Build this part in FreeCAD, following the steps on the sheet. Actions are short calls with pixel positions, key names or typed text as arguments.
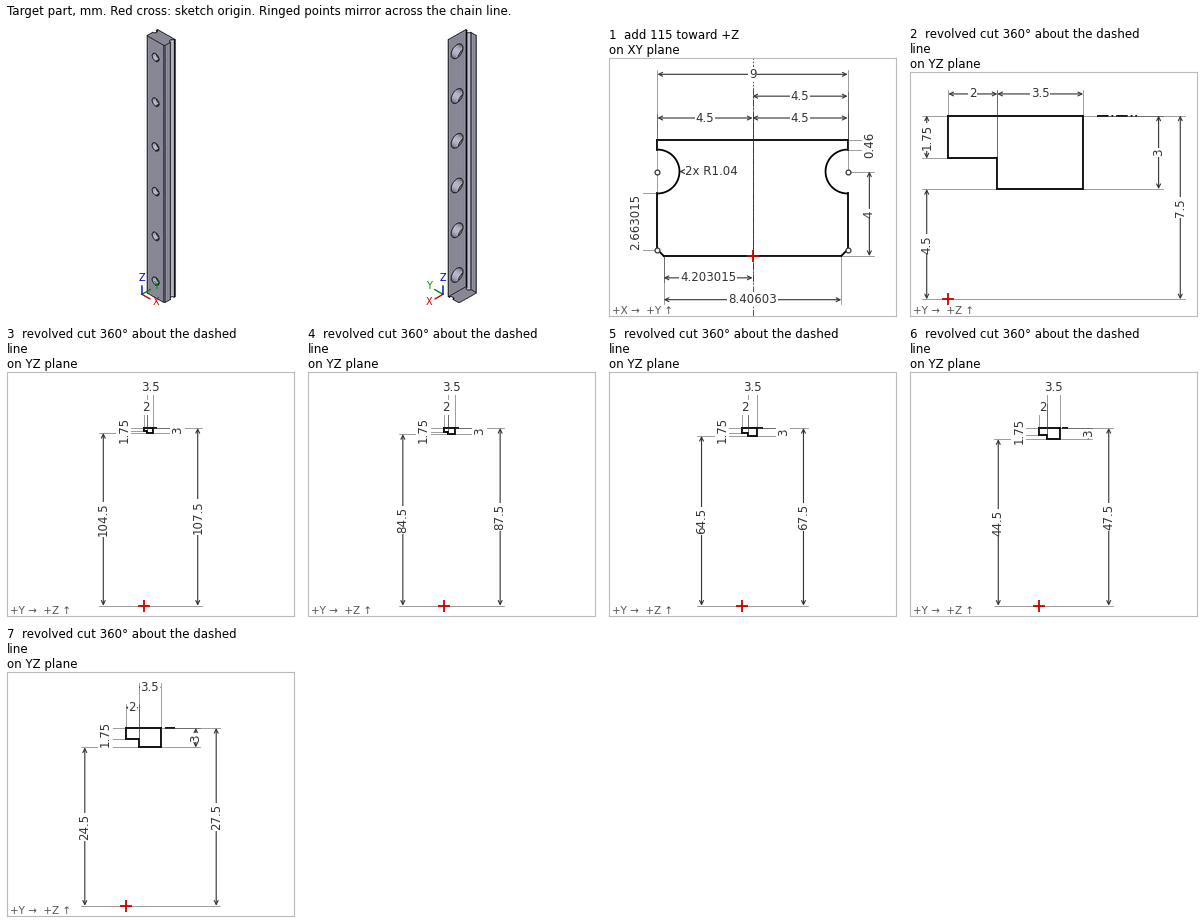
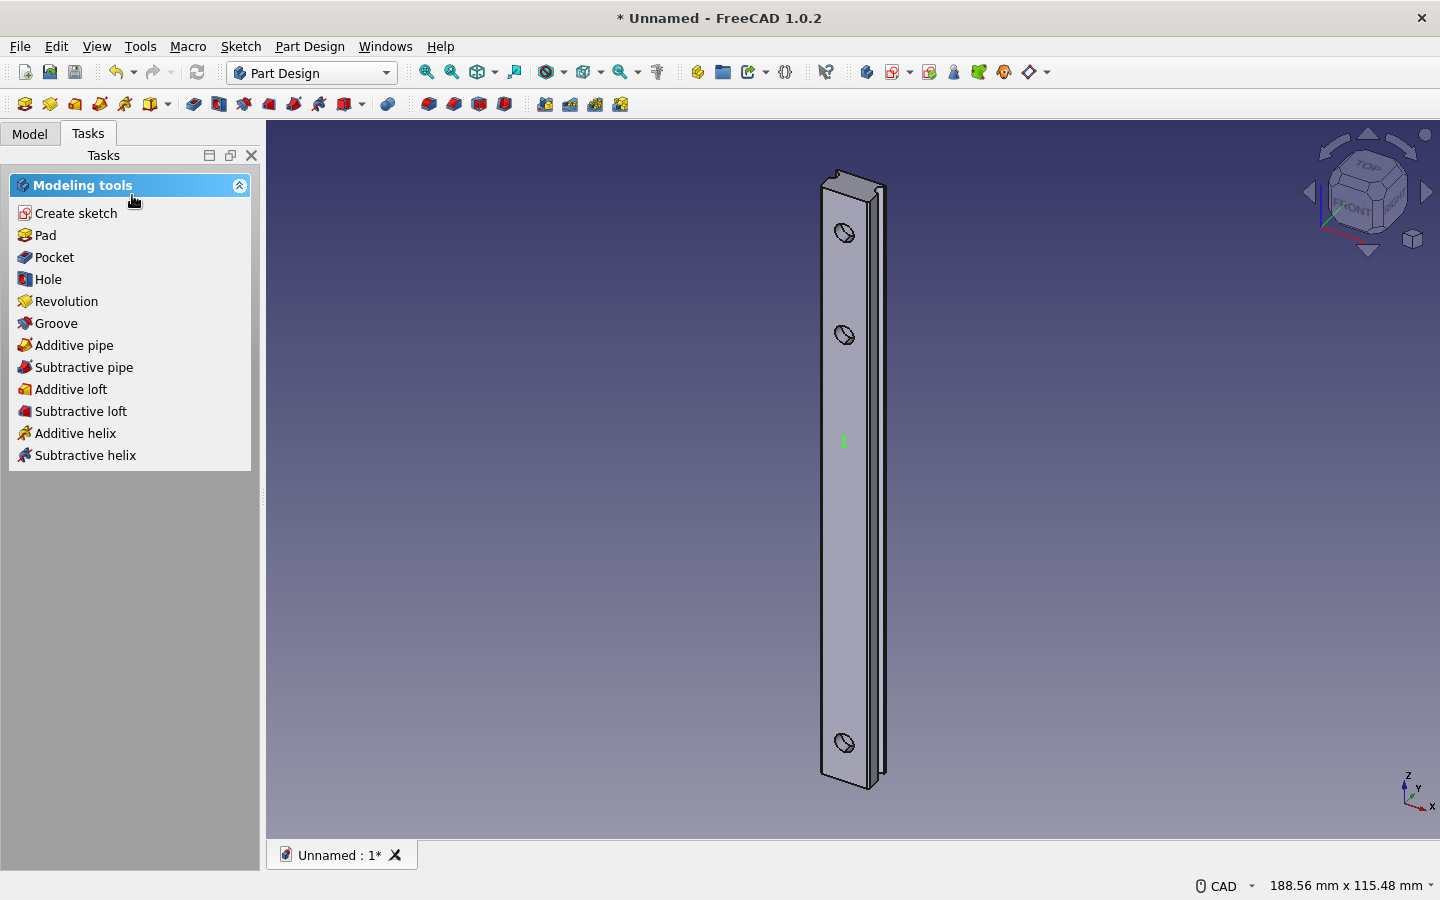
click(244, 104)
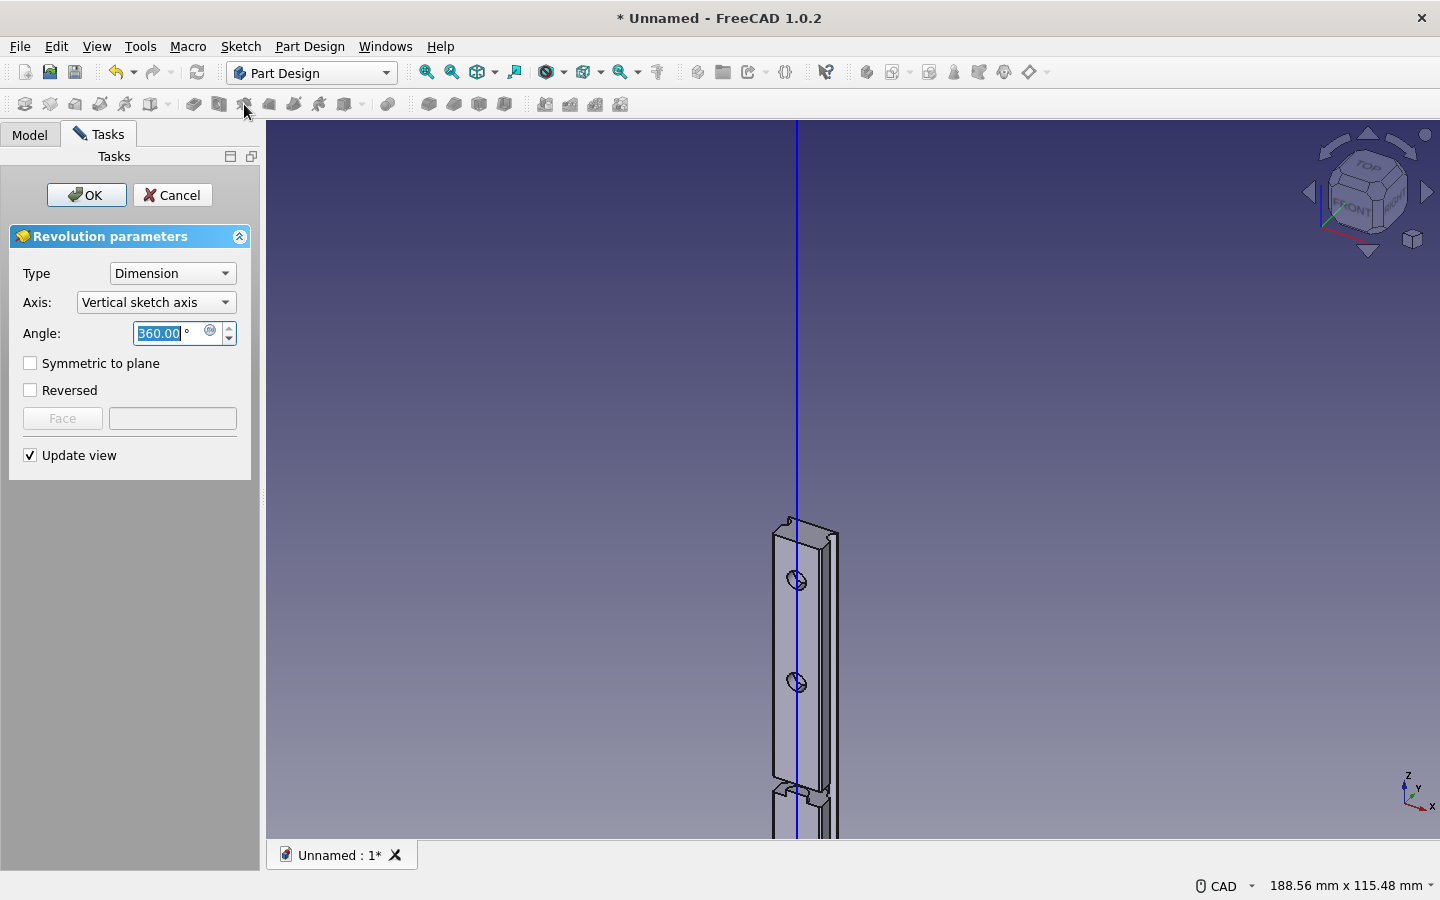
click(157, 302)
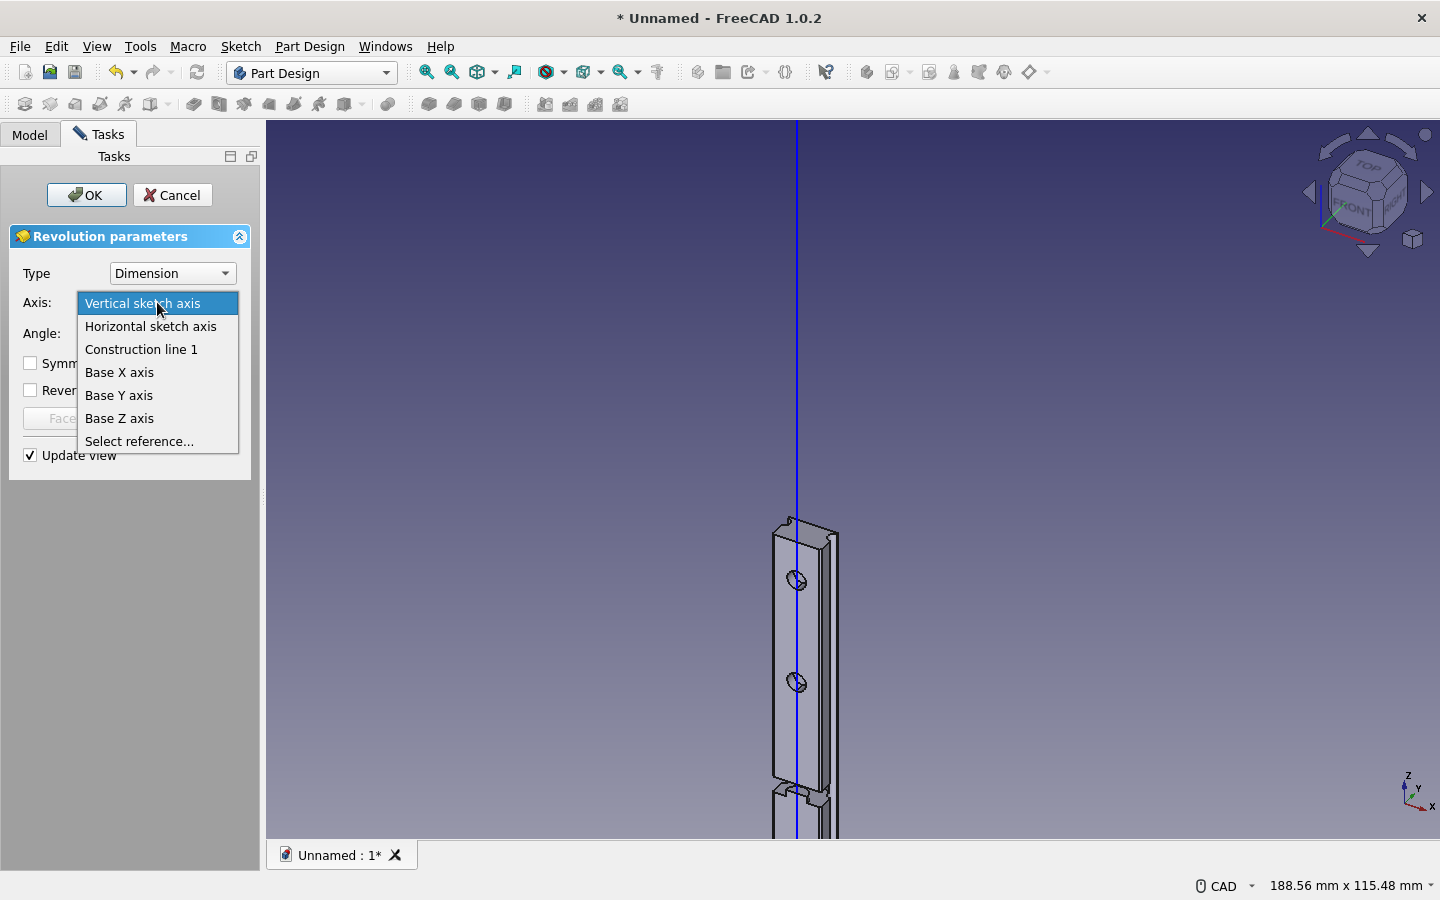
click(156, 350)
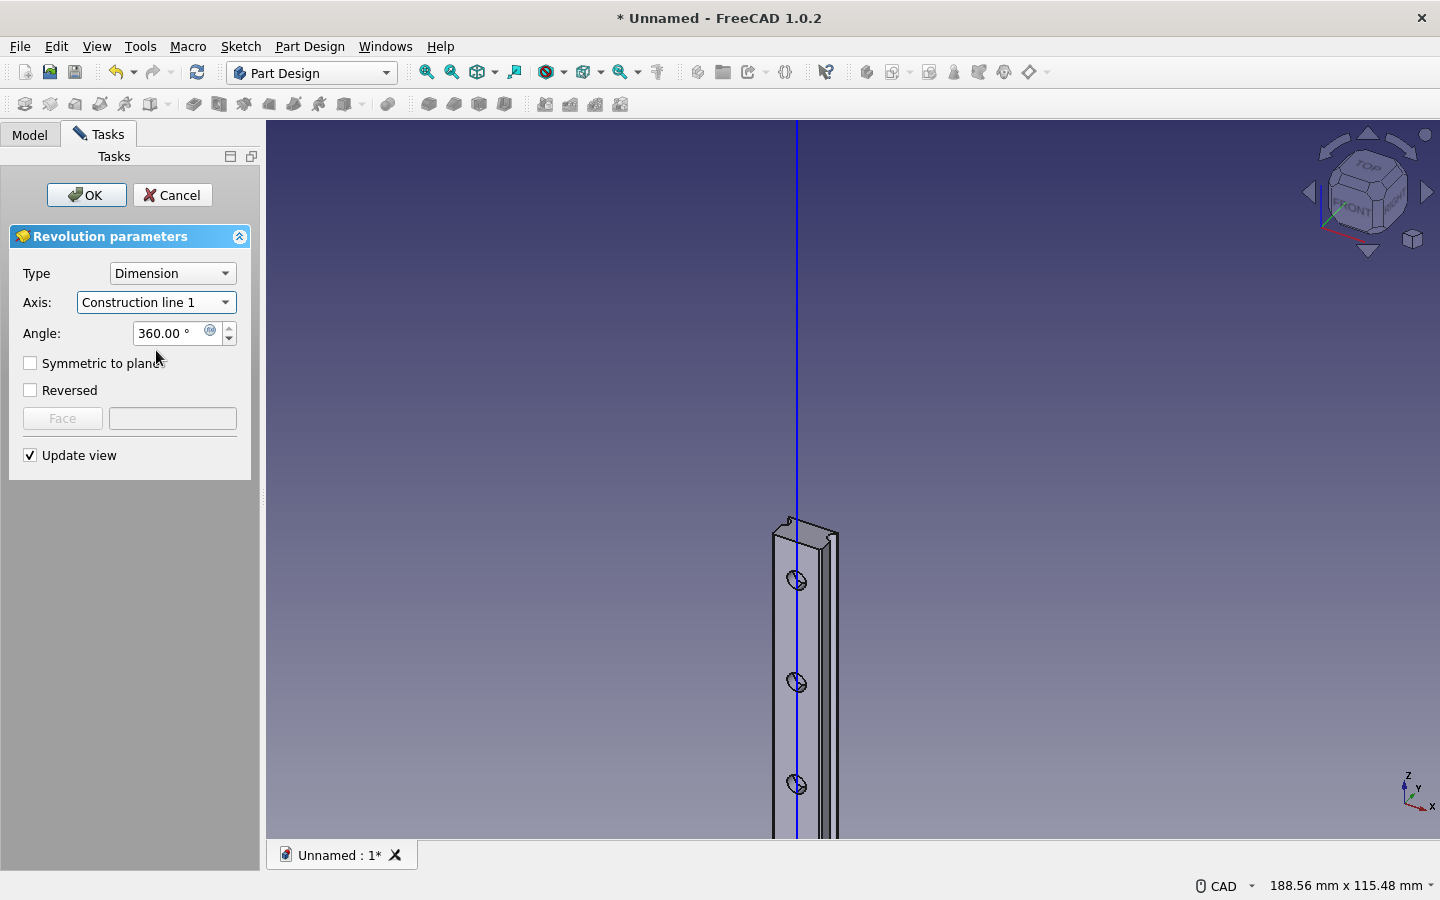
click(87, 195)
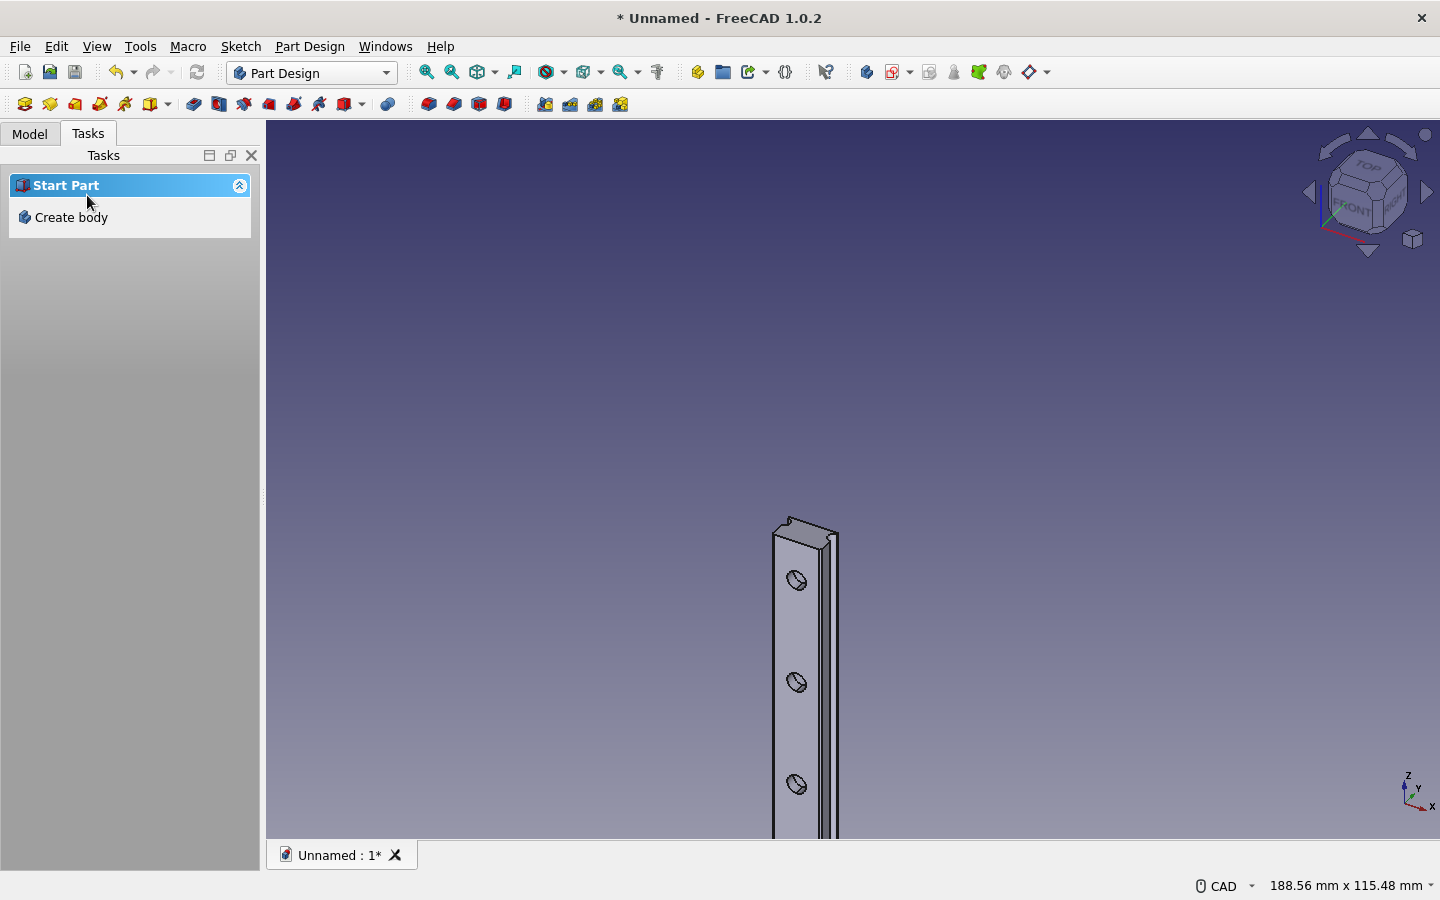
key(v)
key(f)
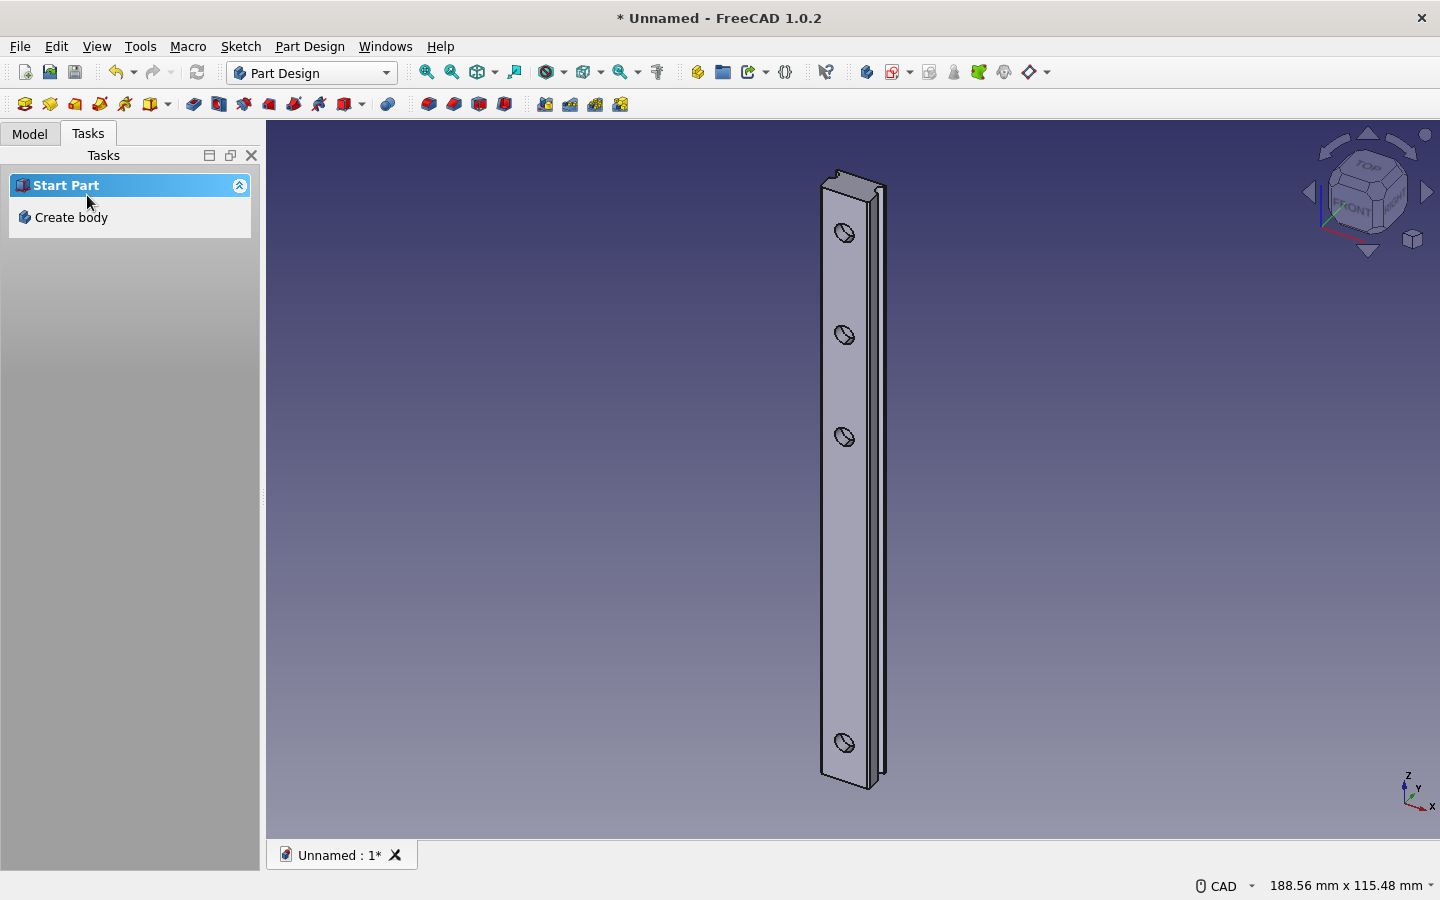
click(892, 72)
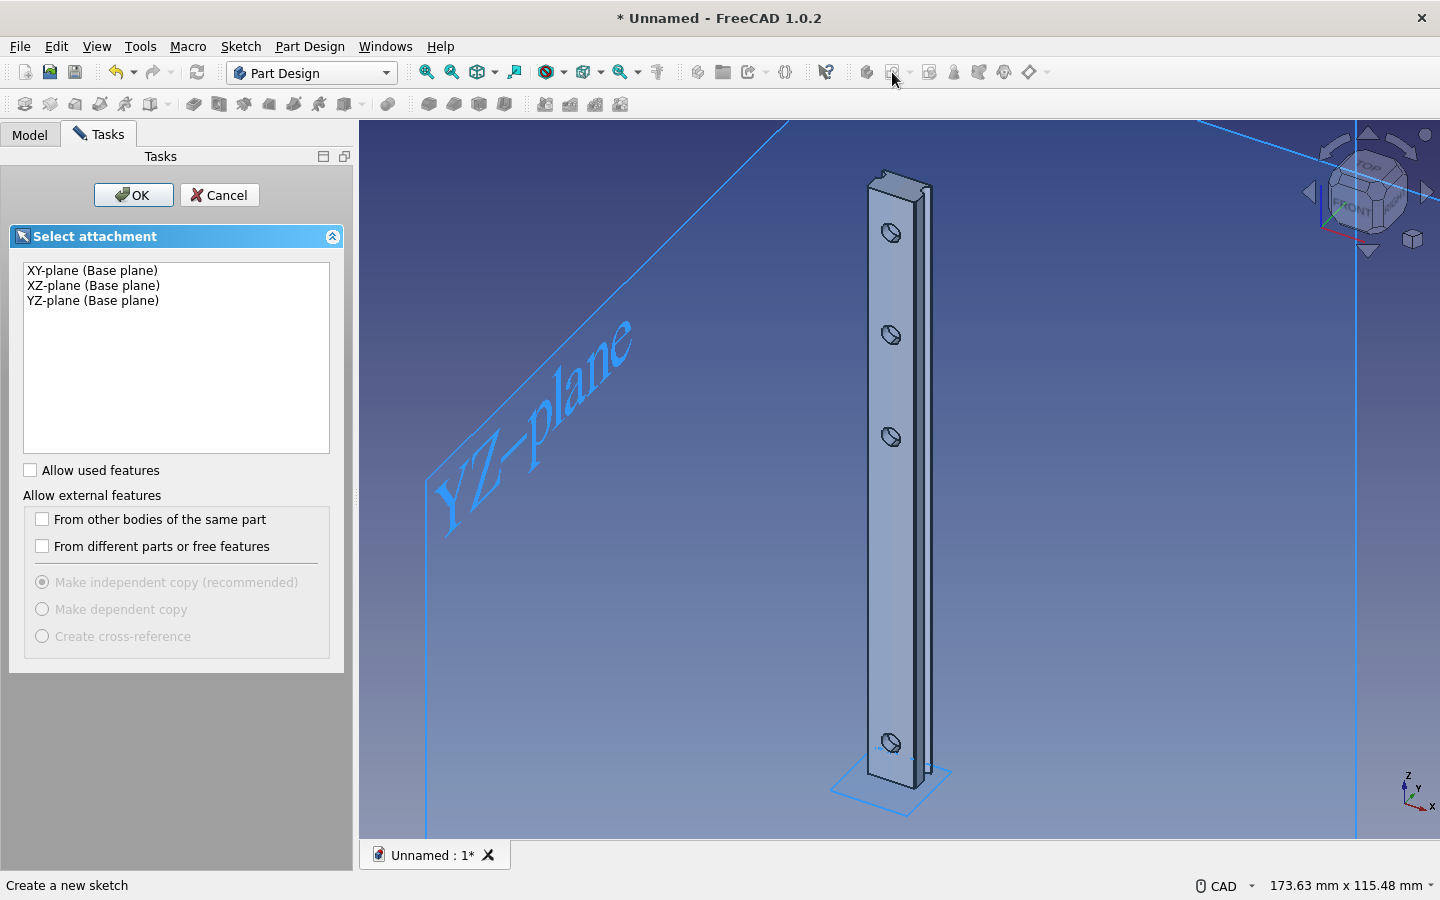
click(84, 300)